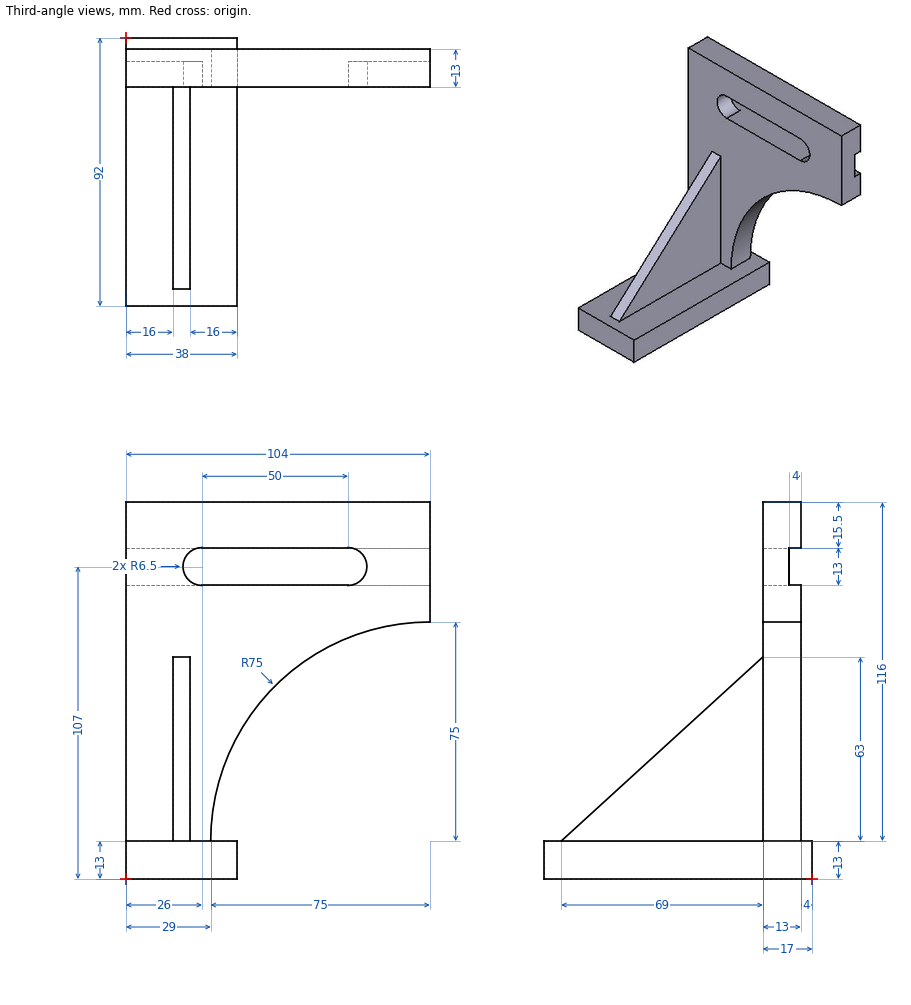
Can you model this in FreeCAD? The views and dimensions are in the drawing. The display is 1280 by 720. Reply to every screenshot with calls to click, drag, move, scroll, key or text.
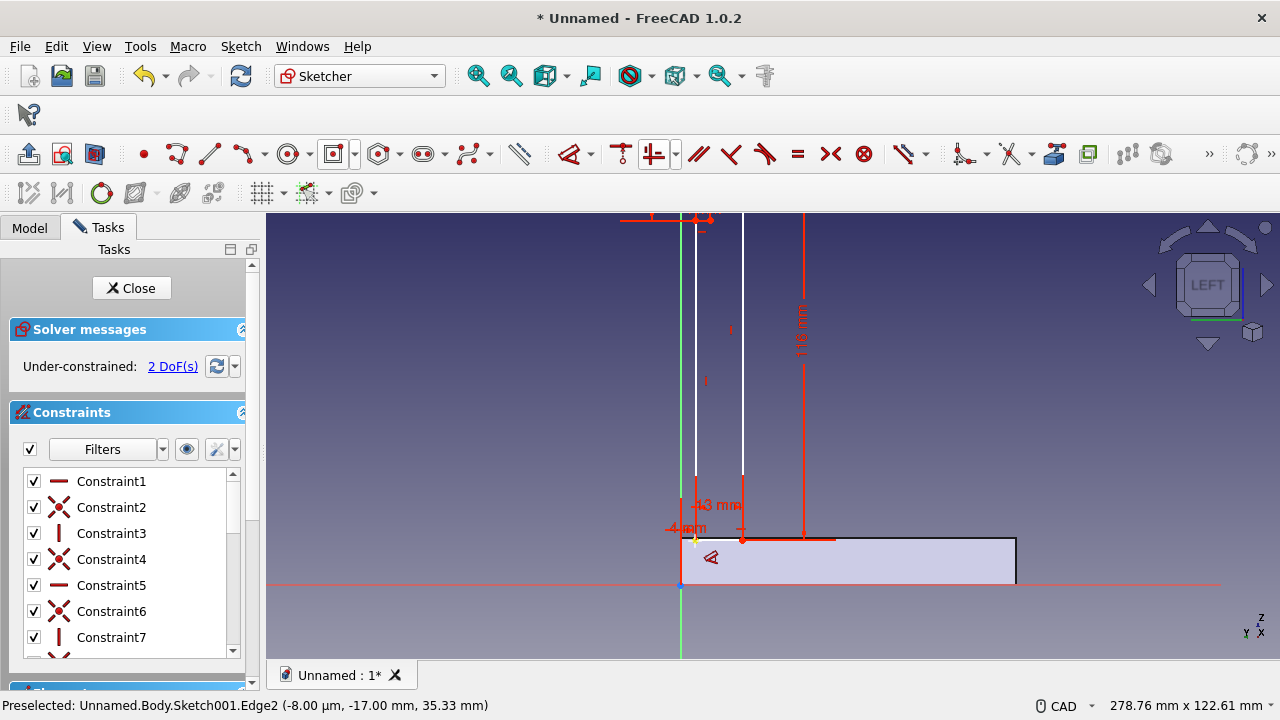
click(696, 540)
click(647, 563)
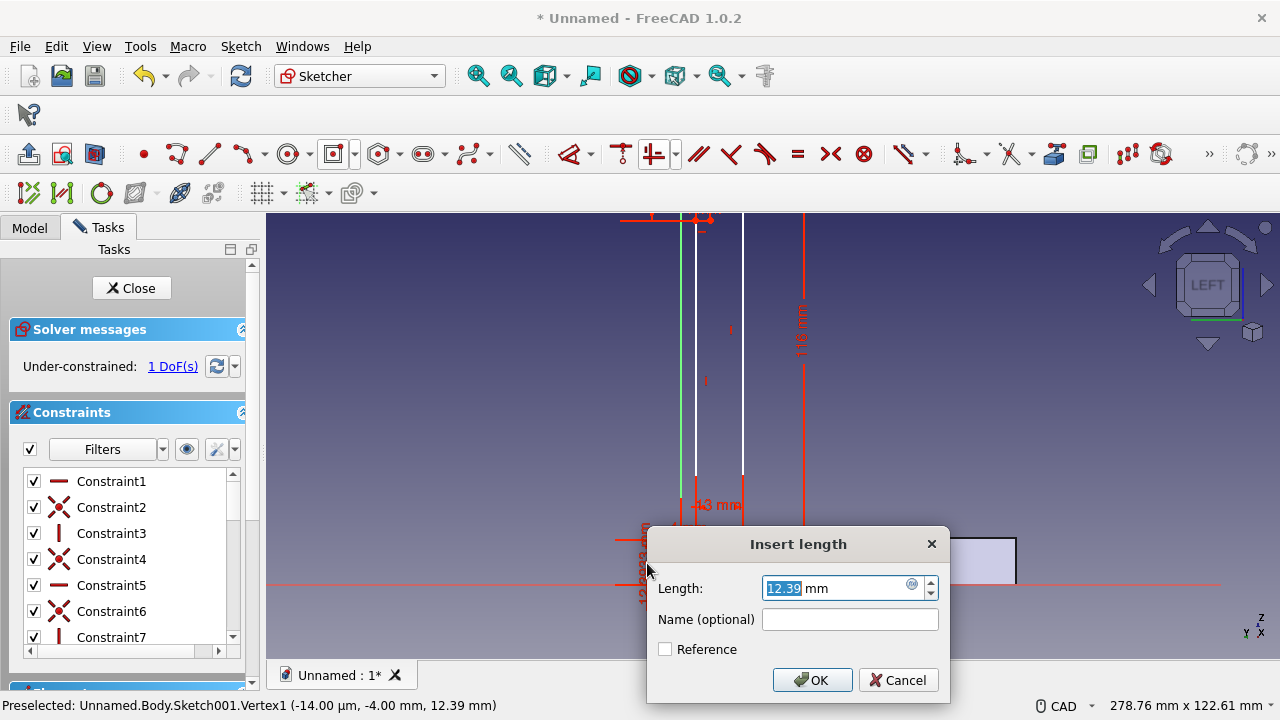
text(13)
key(Return)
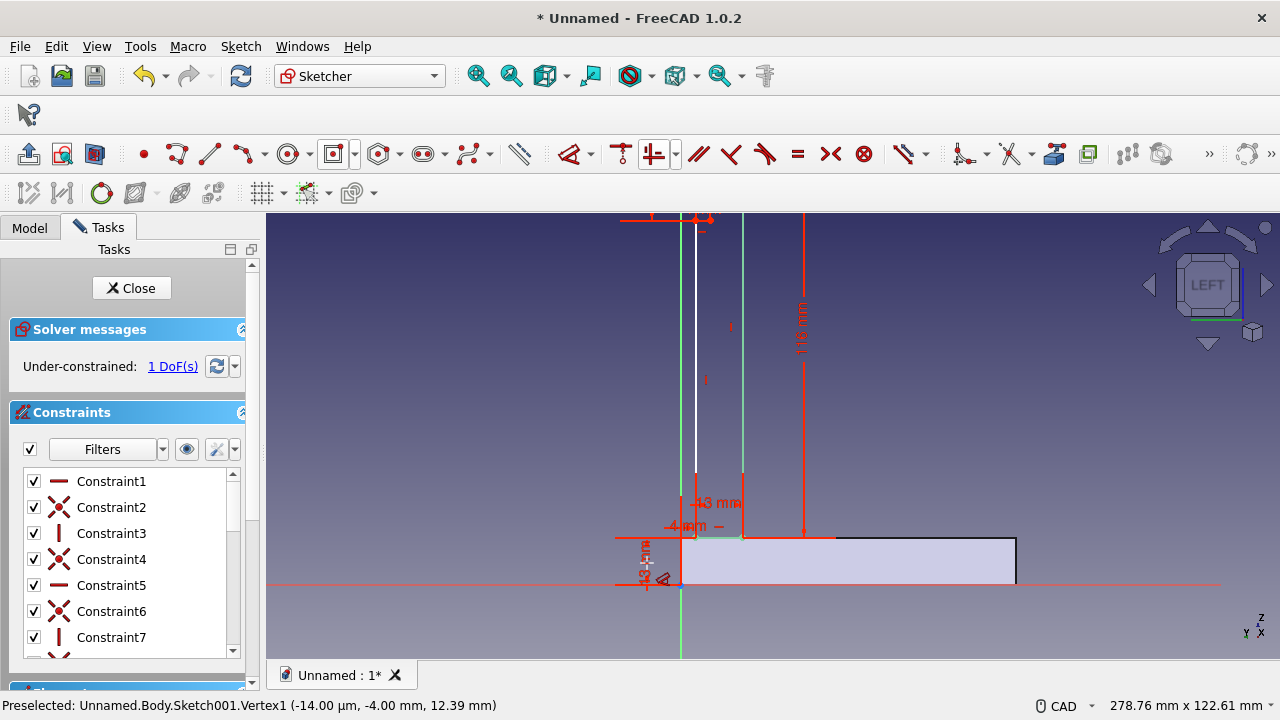
scroll(695, 540, down, 3)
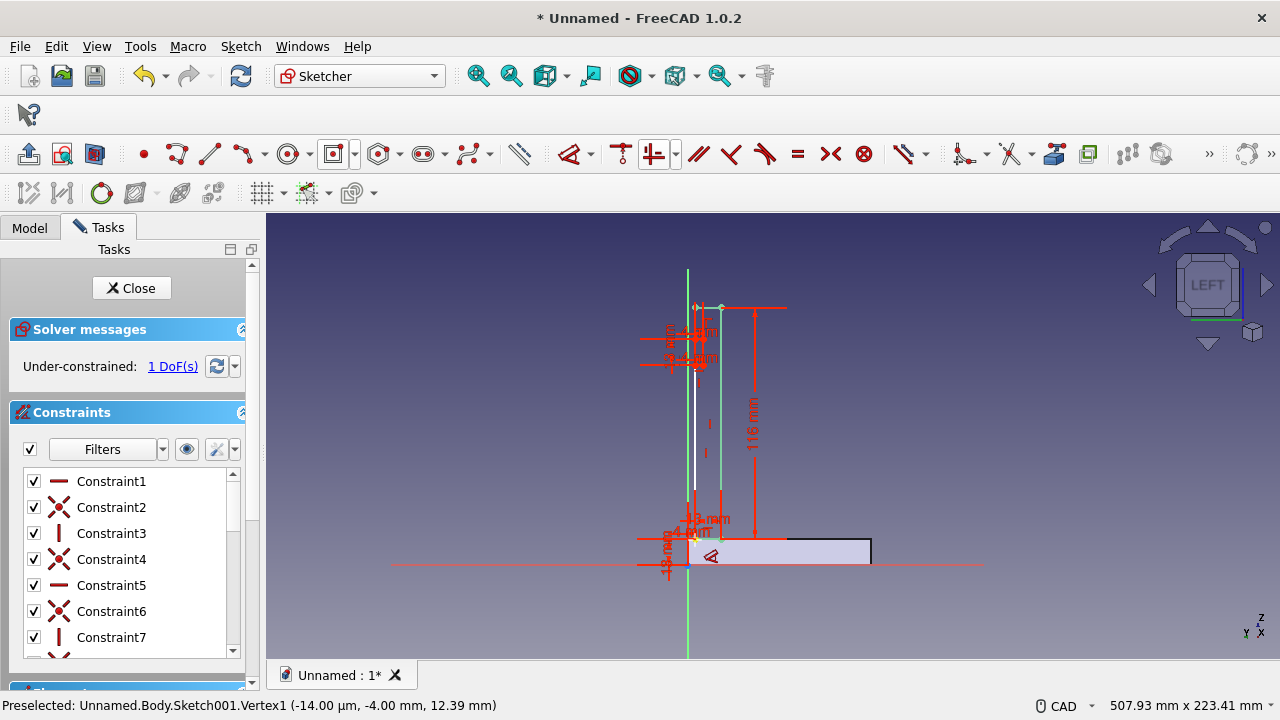
scroll(695, 317, up, 3)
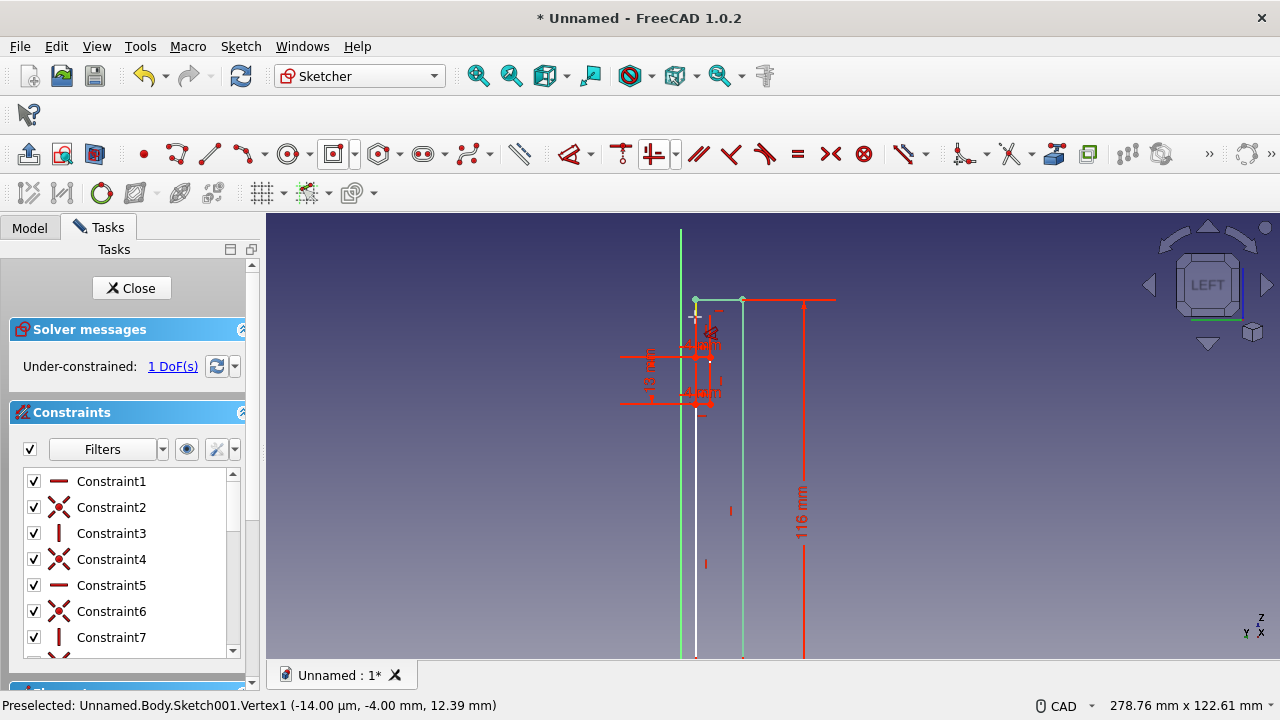
click(696, 317)
click(662, 315)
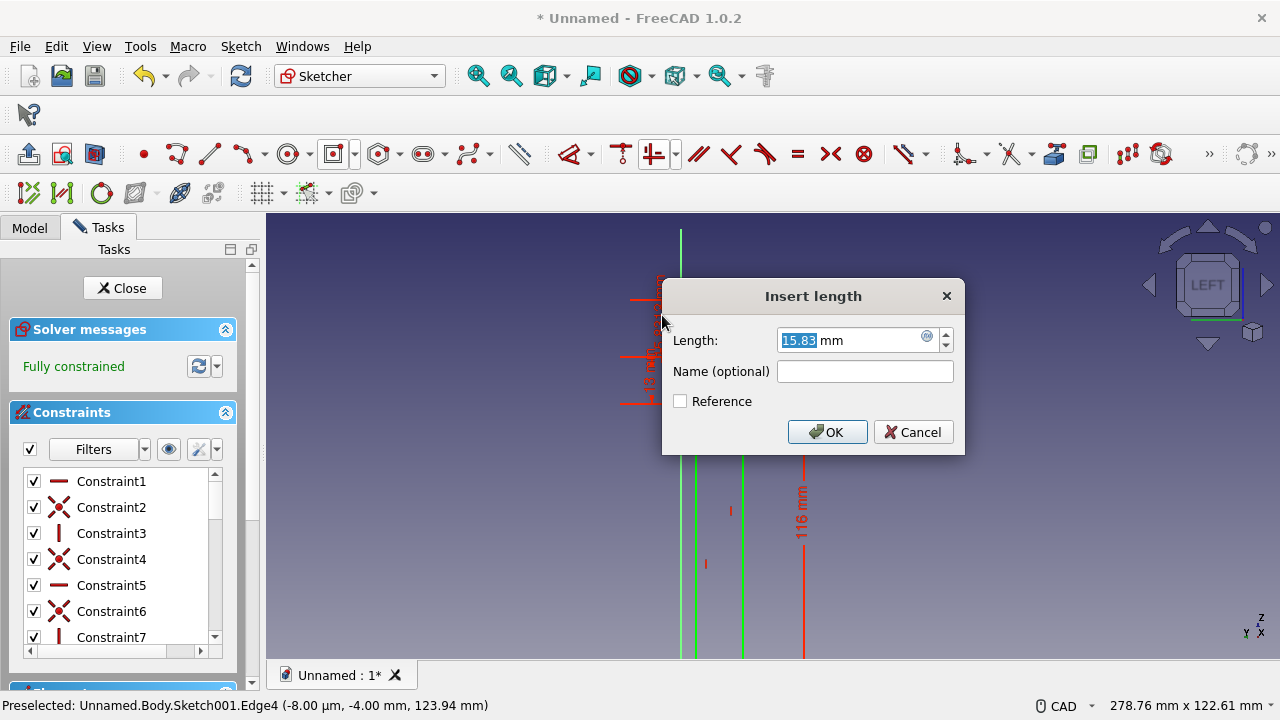
text(15.5)
key(Return)
key(Escape)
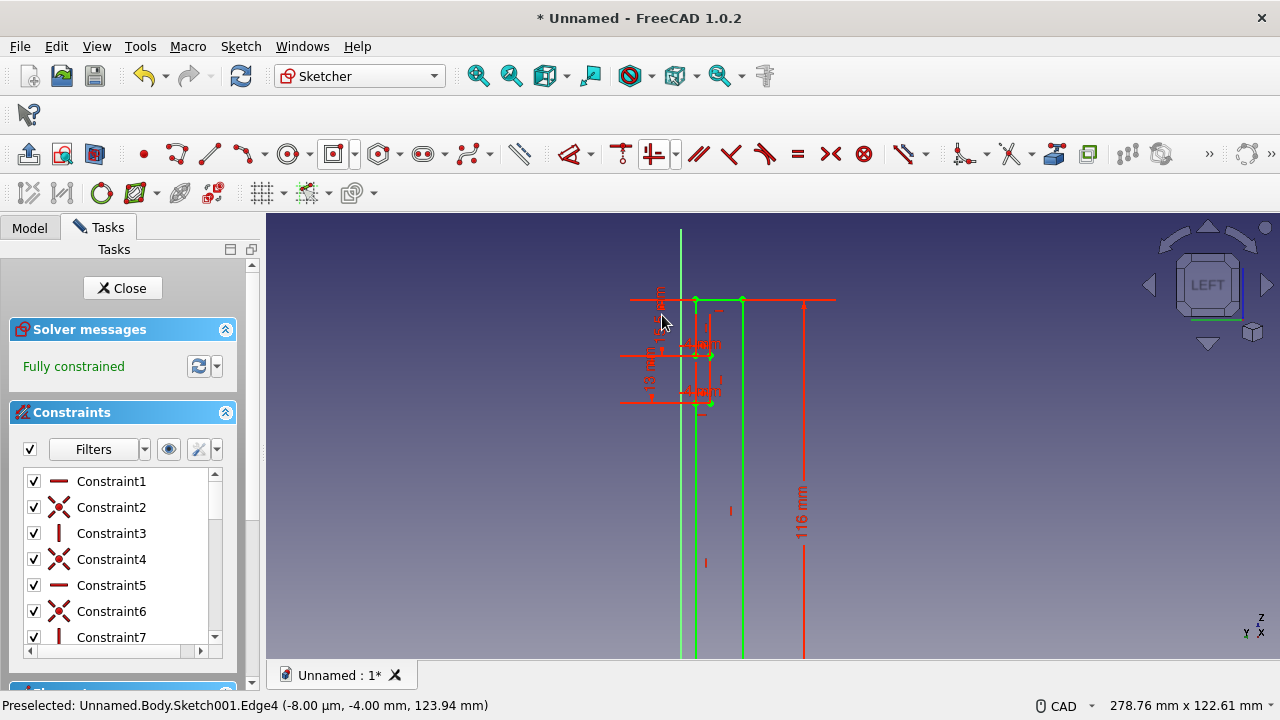
click(123, 288)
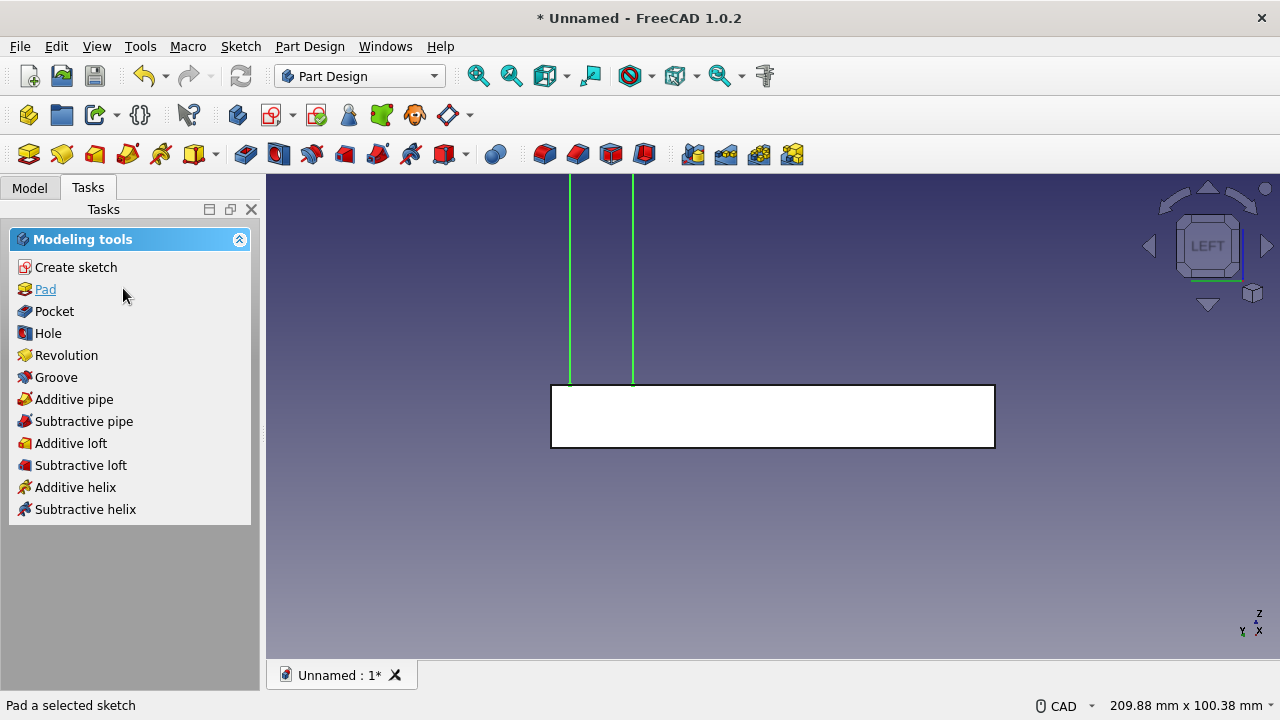
click(29, 154)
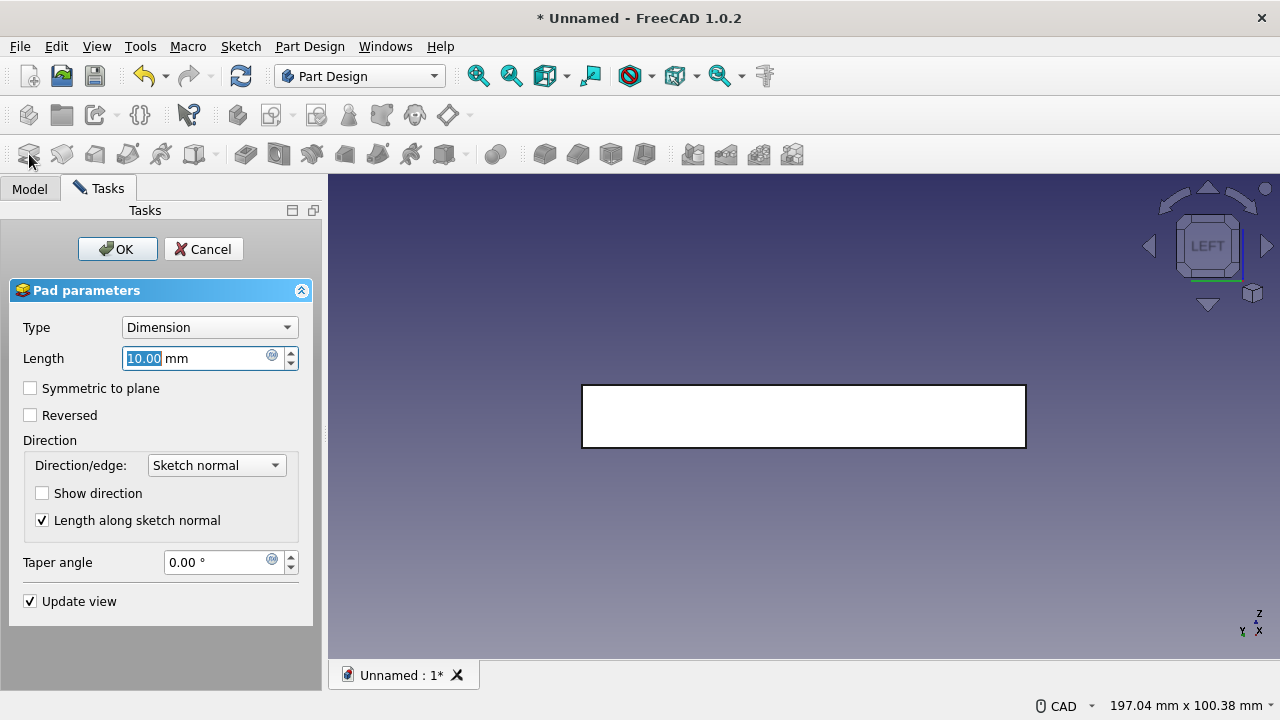
text(104)
key(Tab)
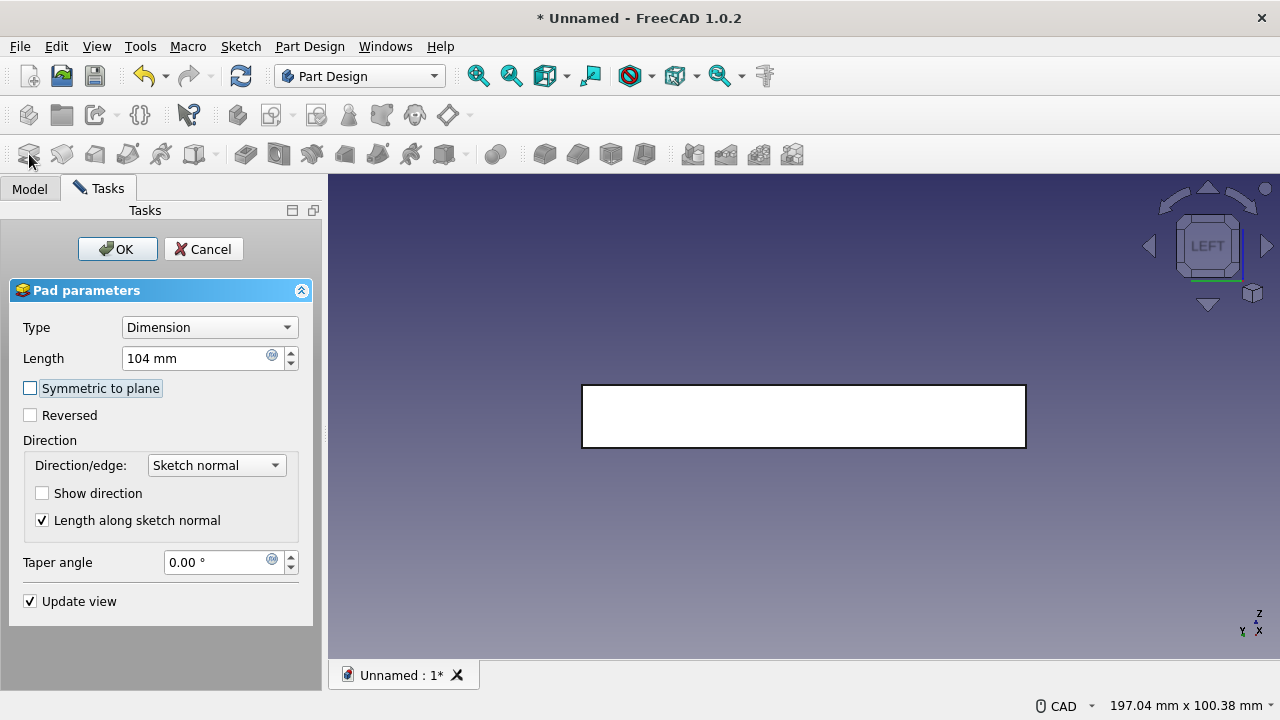
click(31, 415)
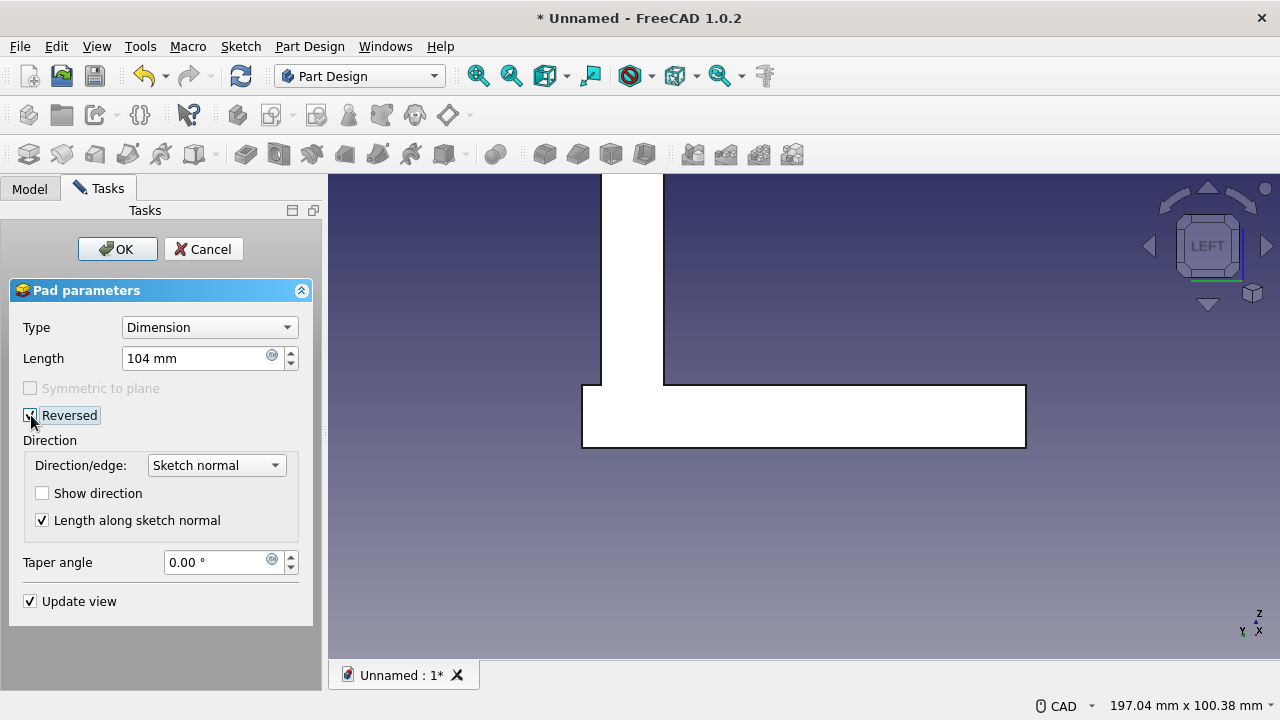
click(118, 249)